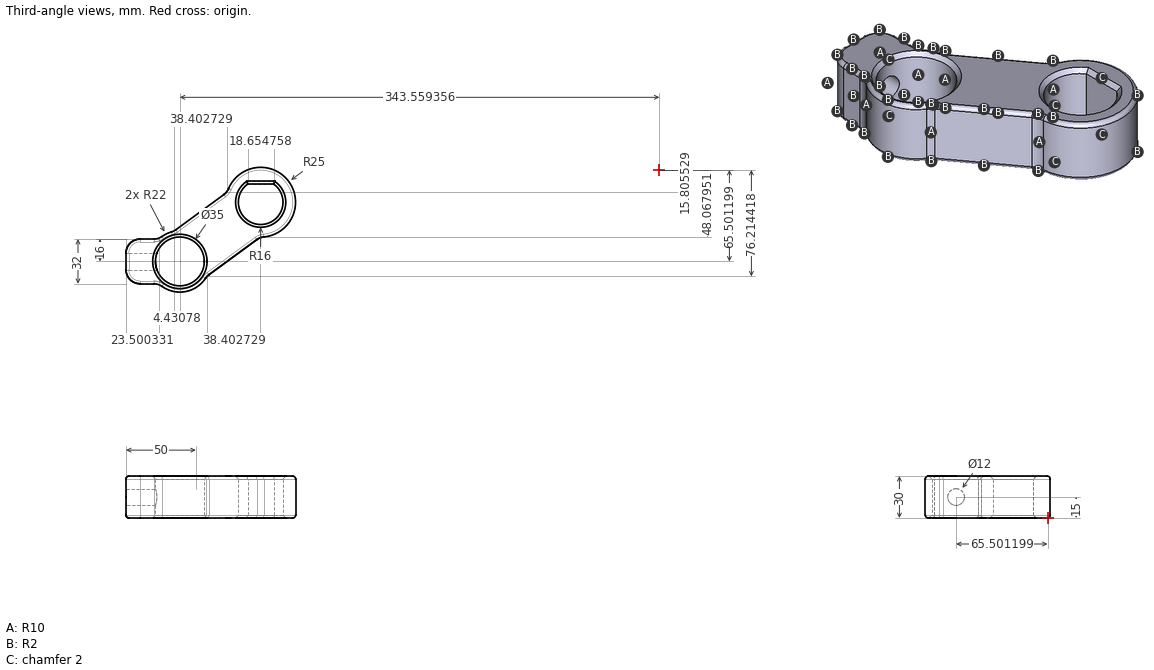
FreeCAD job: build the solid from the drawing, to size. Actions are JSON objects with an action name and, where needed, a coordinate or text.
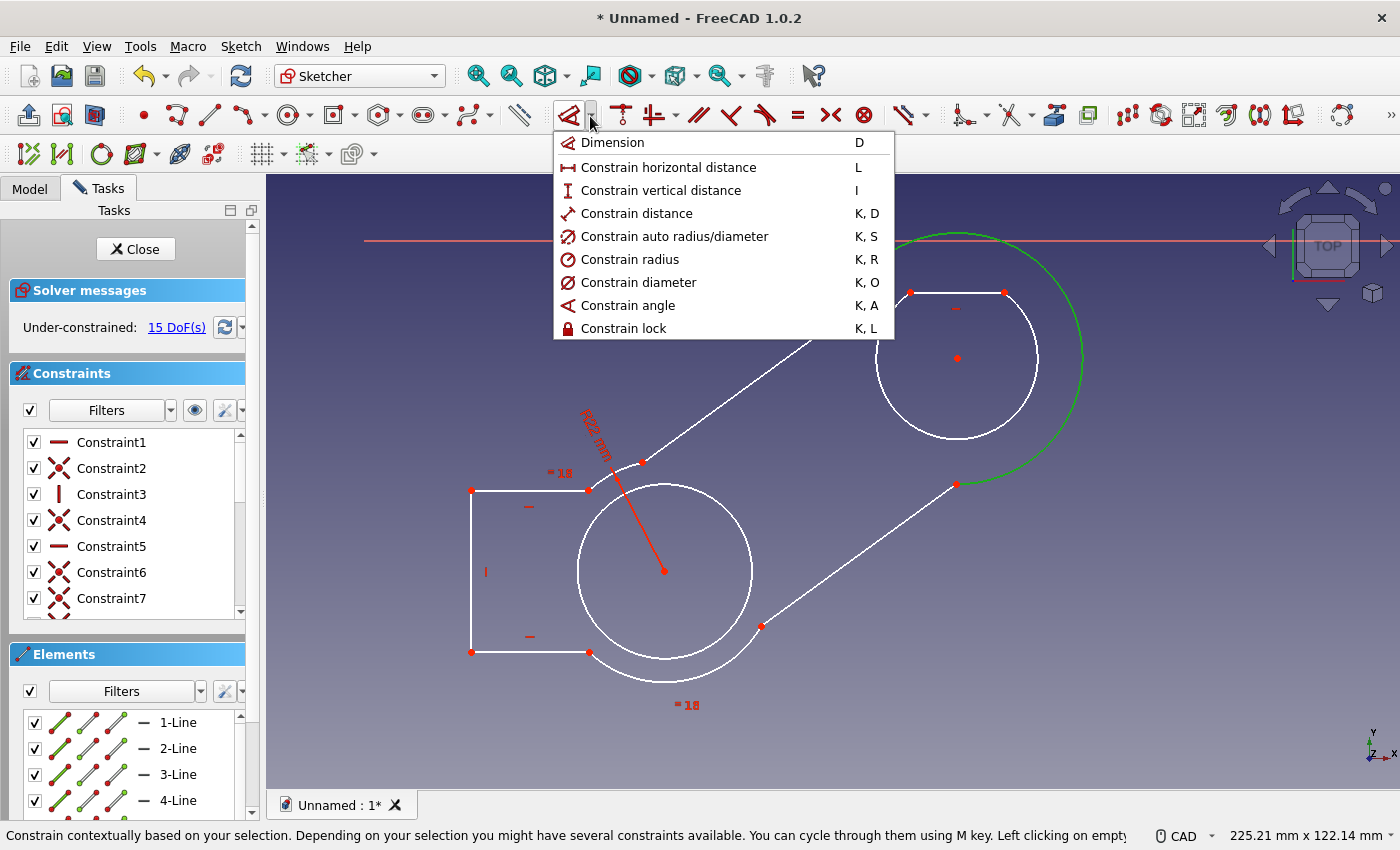
{"action": "left_click", "coordinate": [724, 260]}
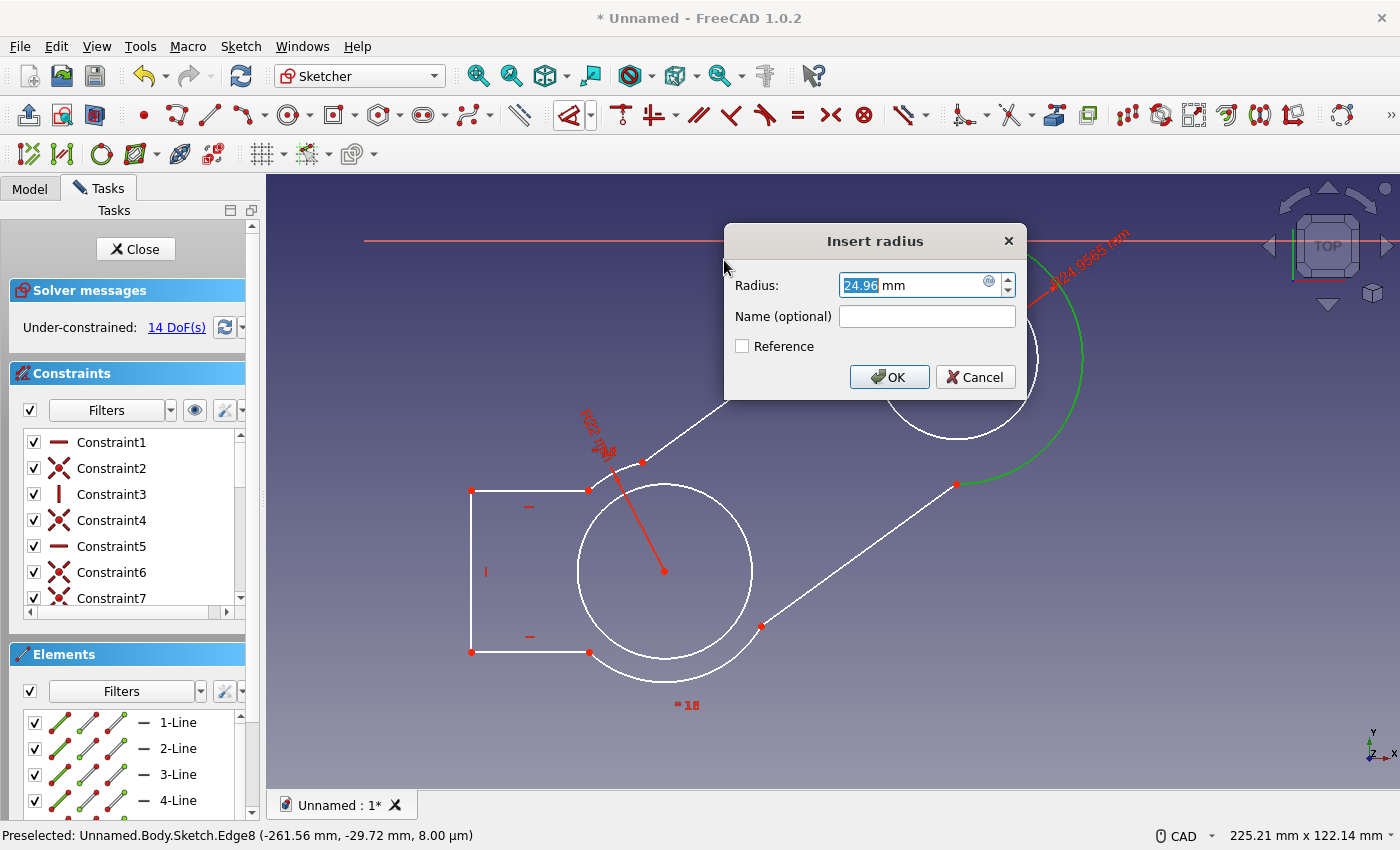
{"action": "type", "text": "25"}
{"action": "key", "text": "Return"}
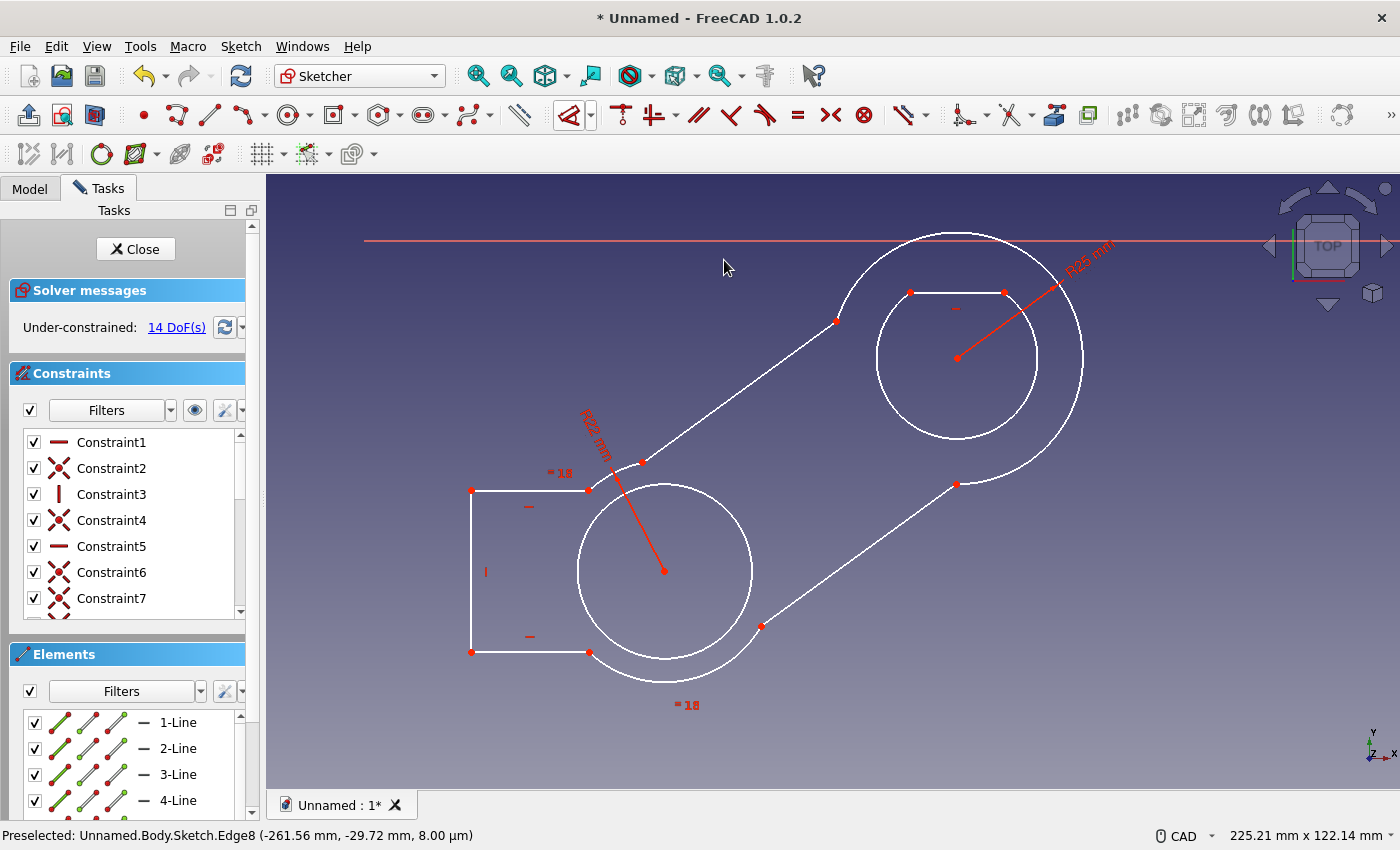
{"action": "left_click", "coordinate": [889, 401]}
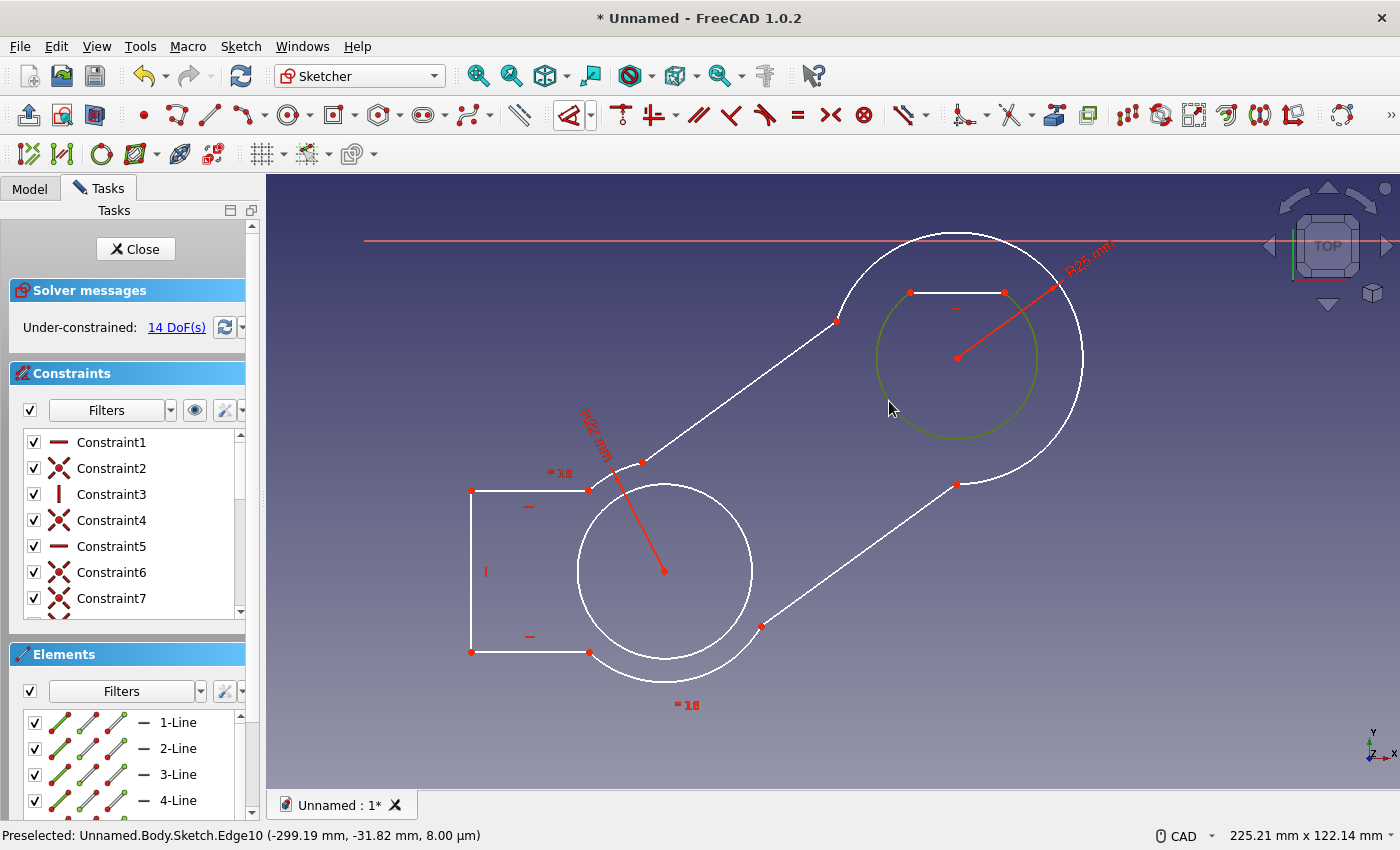
{"action": "left_click", "coordinate": [590, 116]}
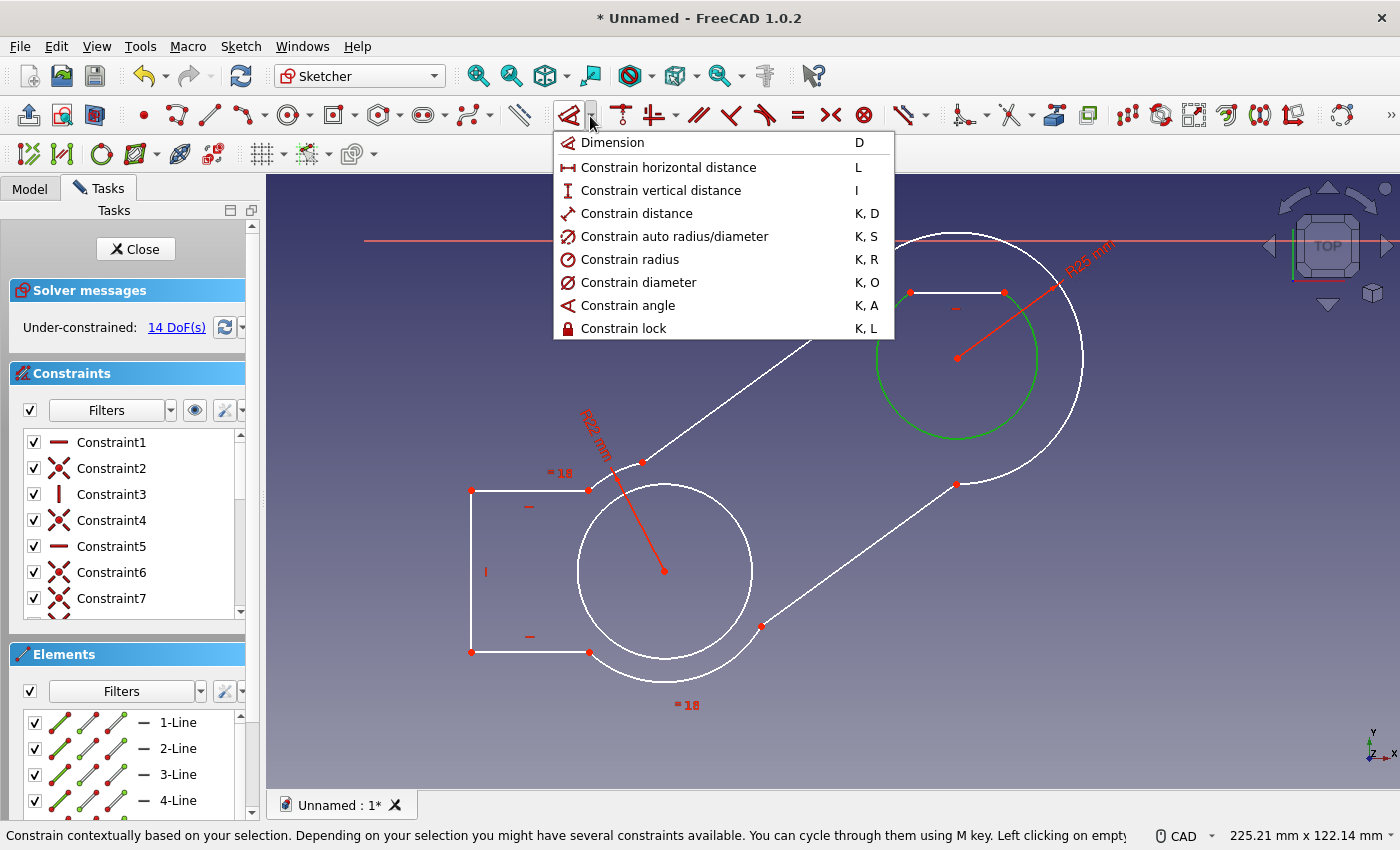
{"action": "left_click", "coordinate": [724, 260]}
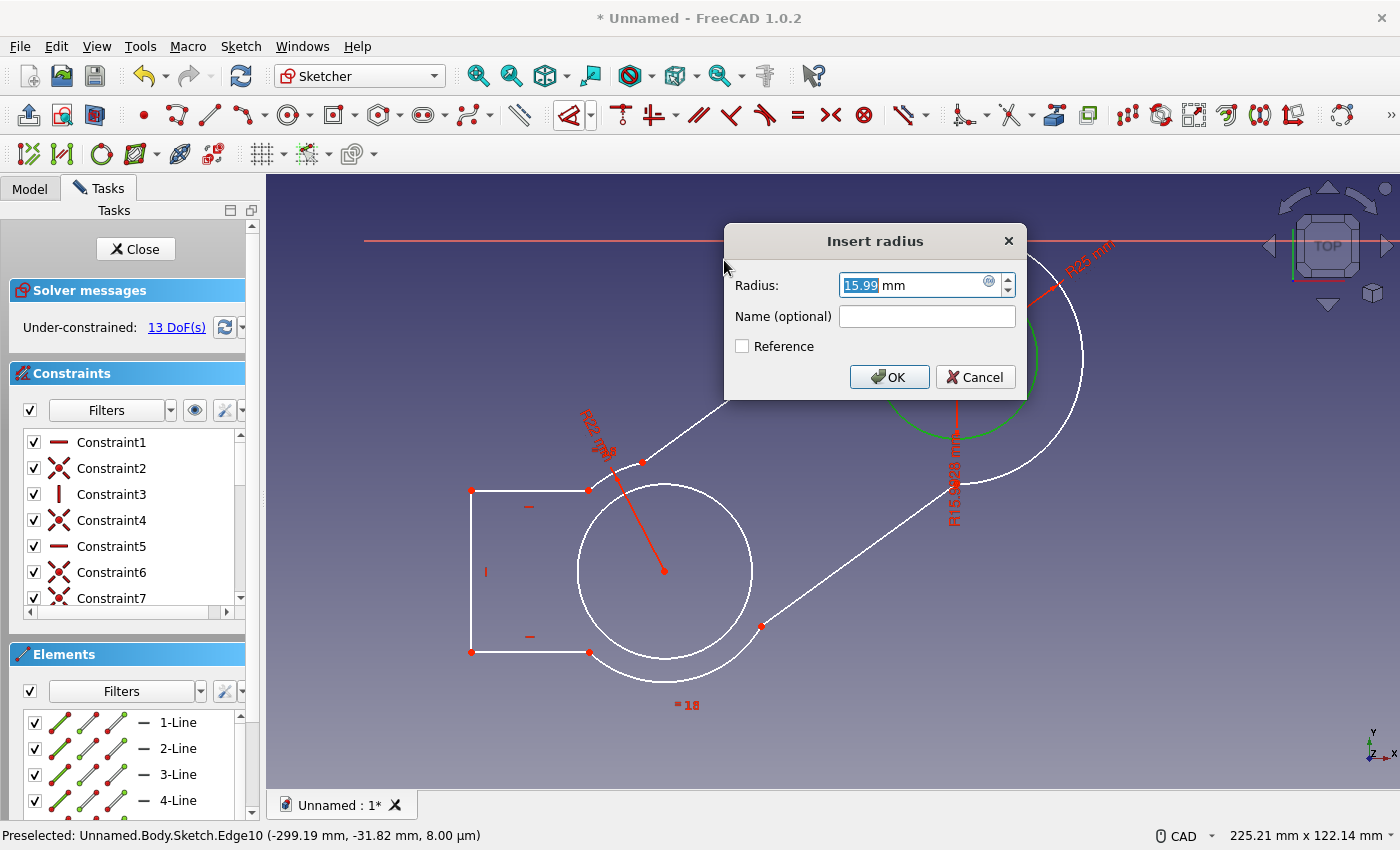
{"action": "type", "text": "16"}
{"action": "key", "text": "Return"}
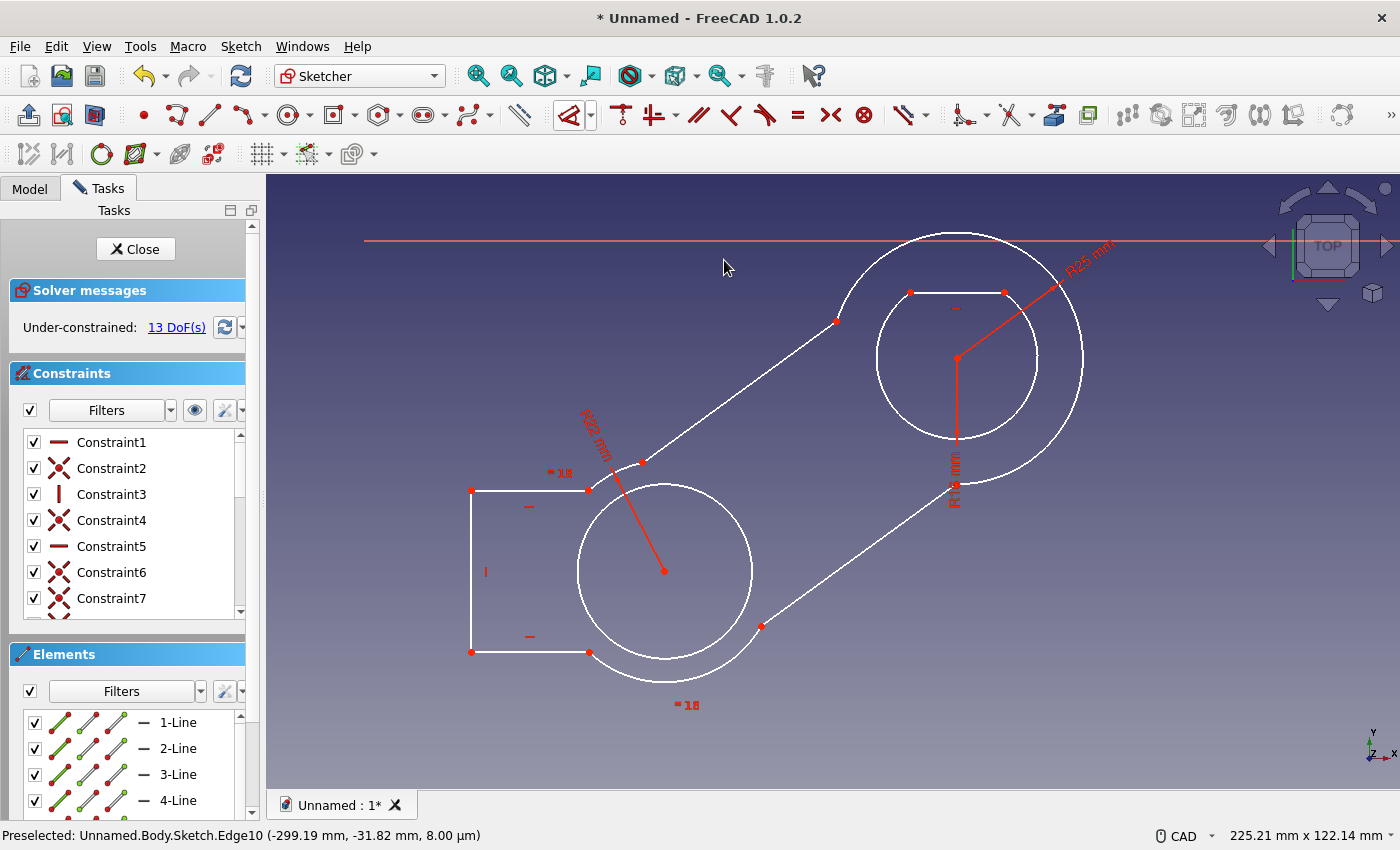
{"action": "left_click", "coordinate": [726, 510]}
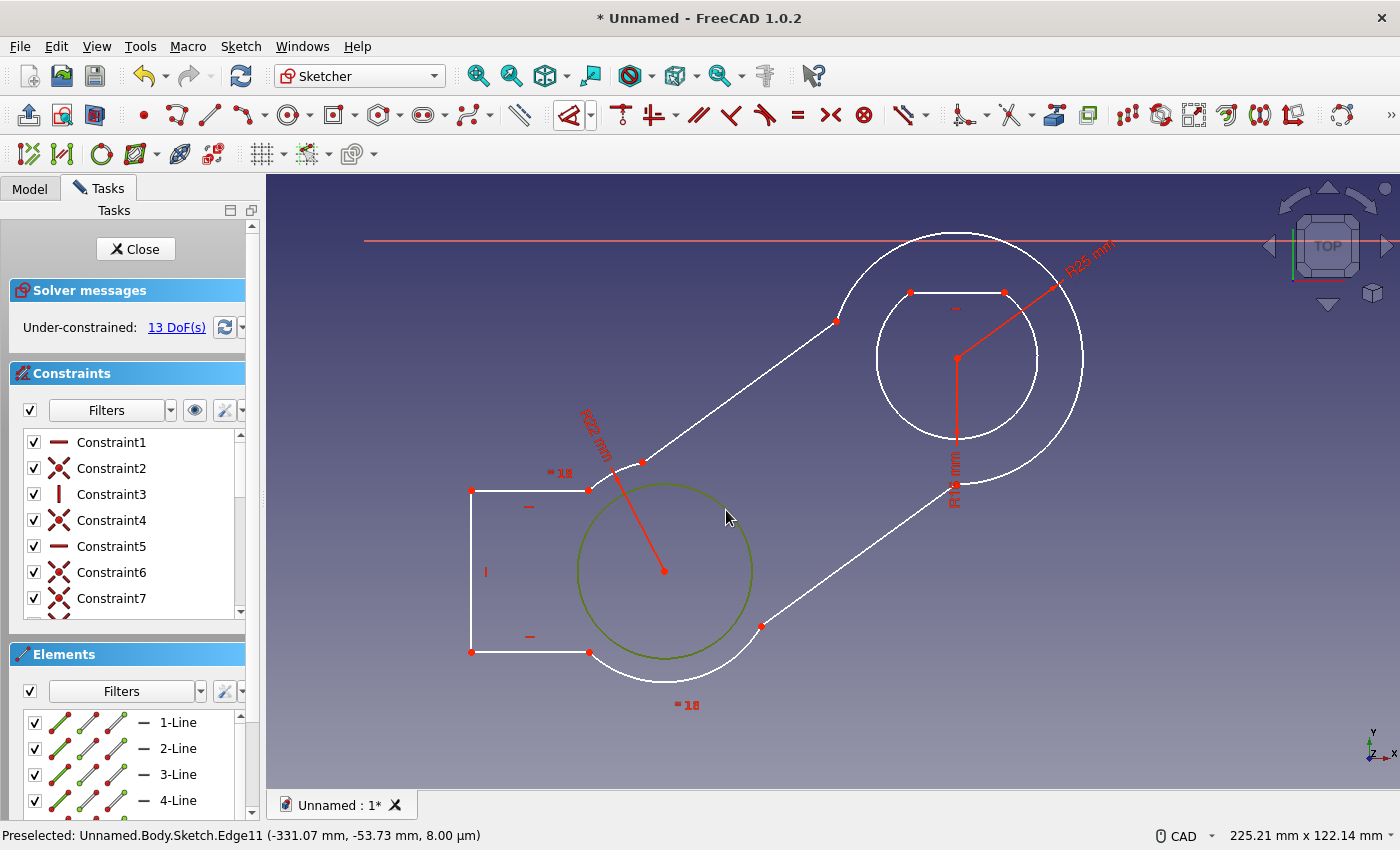
{"action": "key", "text": "k o"}